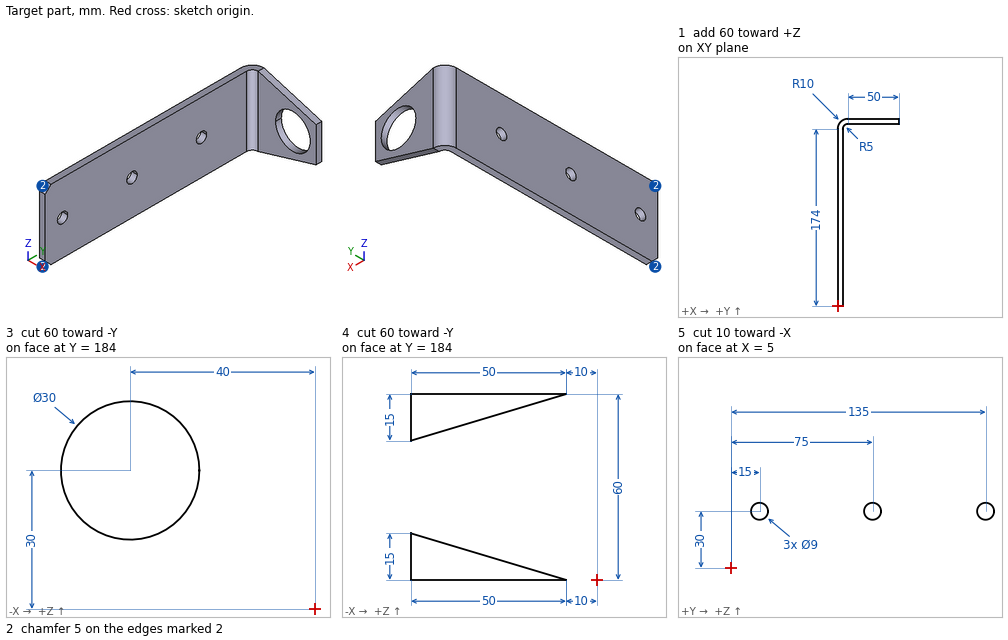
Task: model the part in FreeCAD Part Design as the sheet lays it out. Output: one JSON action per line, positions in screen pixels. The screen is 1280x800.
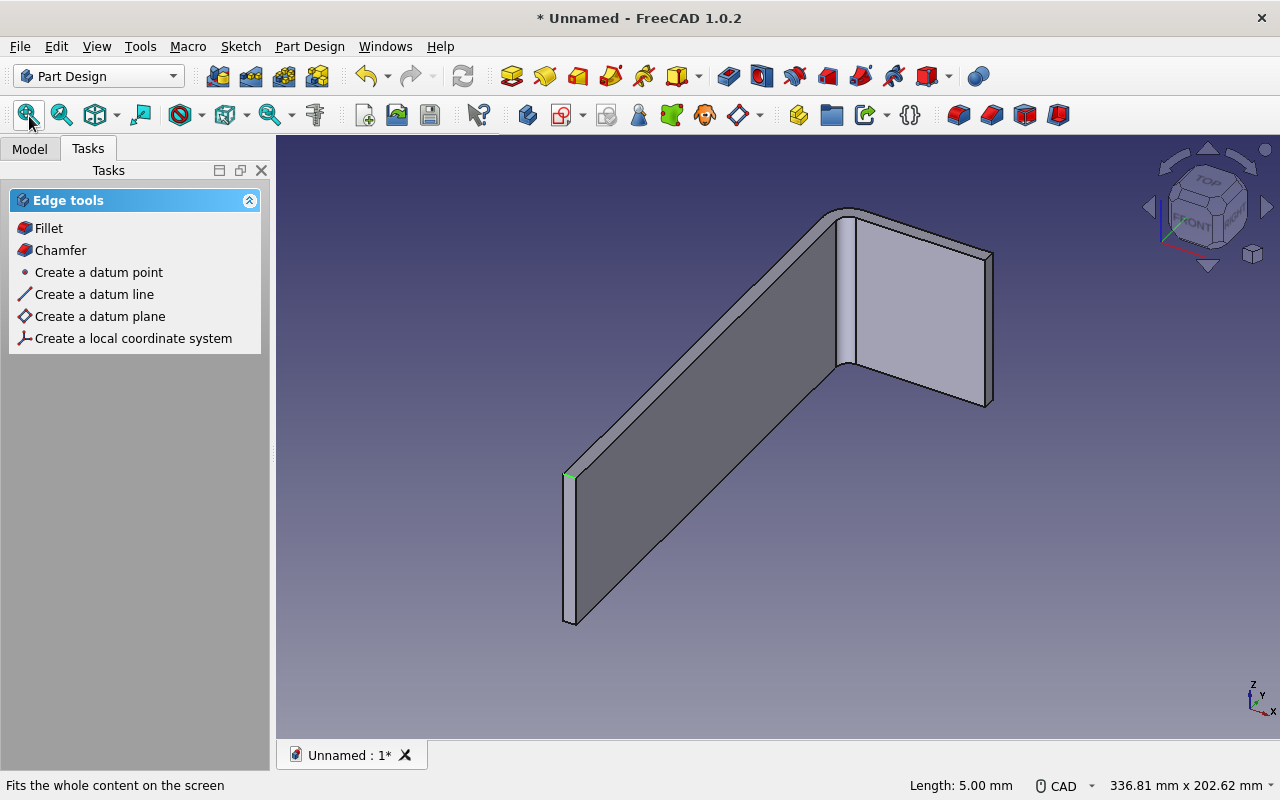
{"action": "key", "text": "0"}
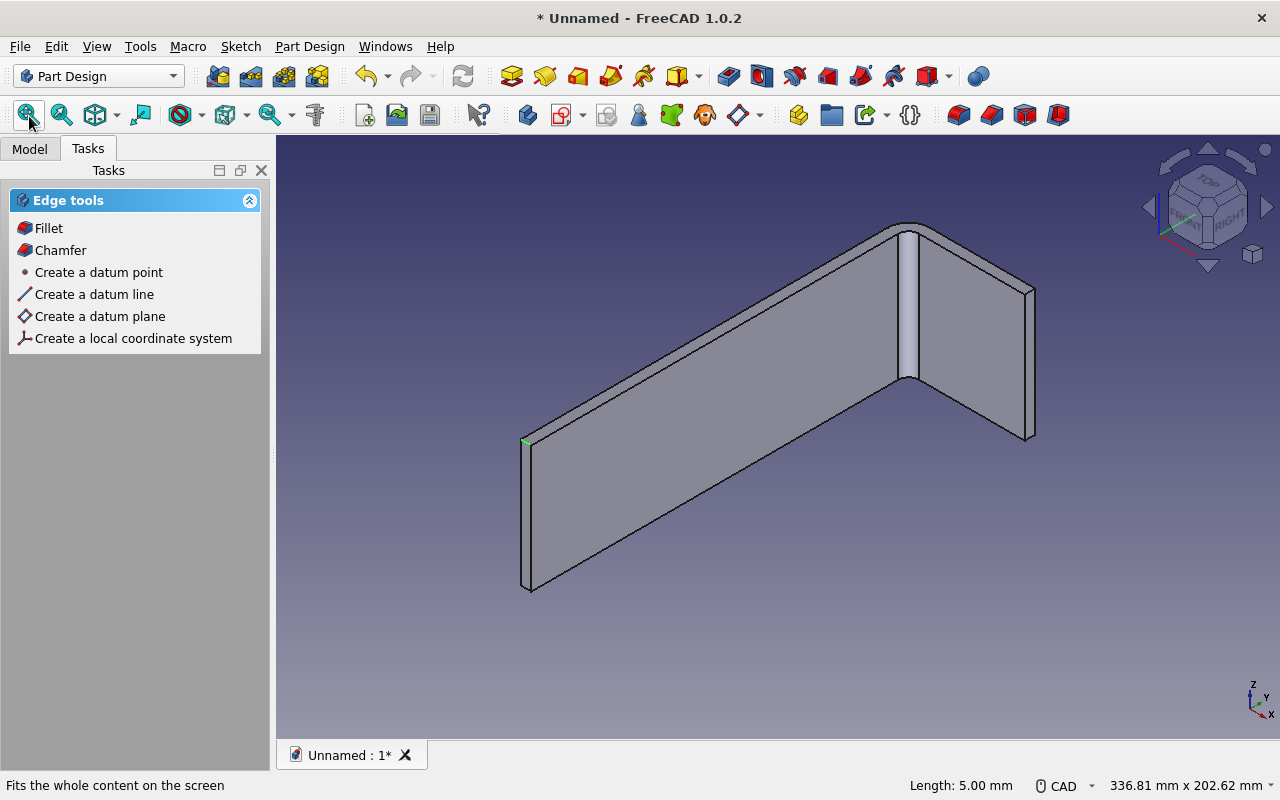
{"action": "scroll", "coordinate": [526, 588], "scroll_direction": "up", "scroll_amount": 5}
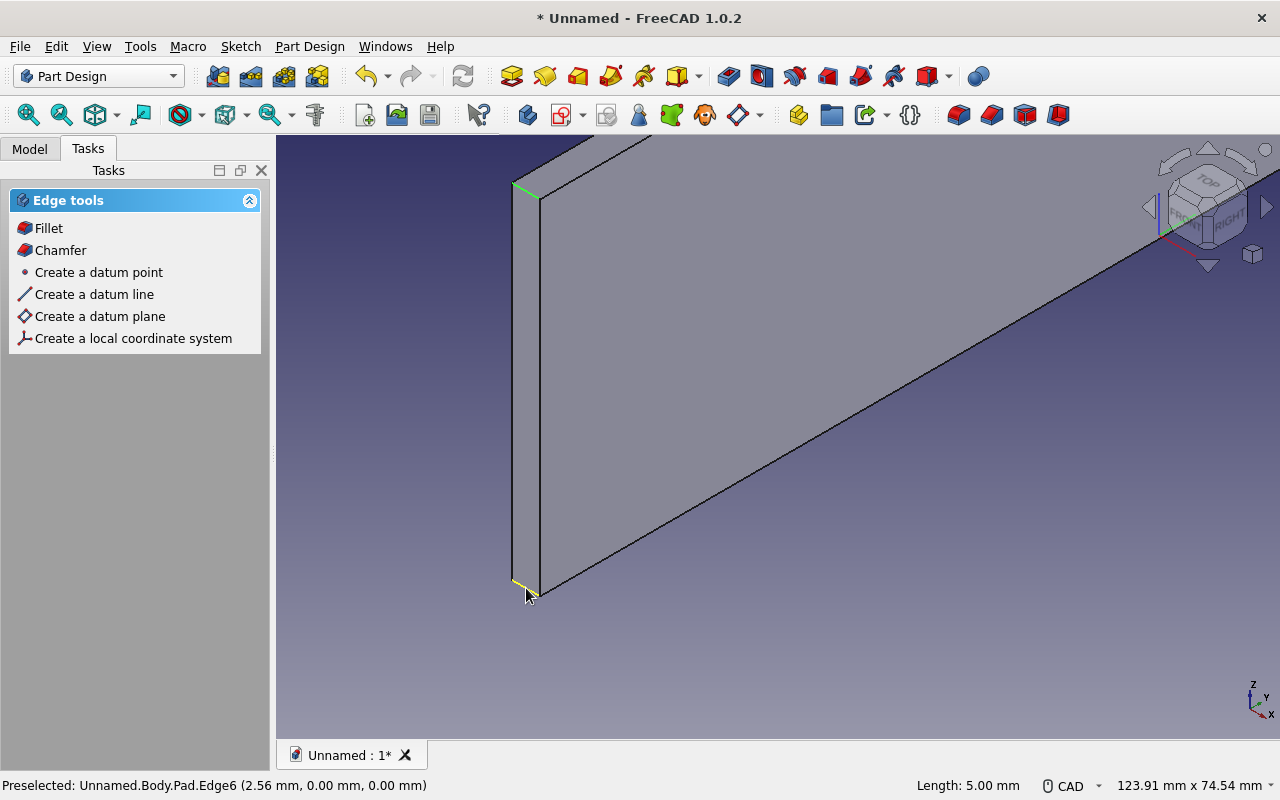
{"action": "key", "text": "v f"}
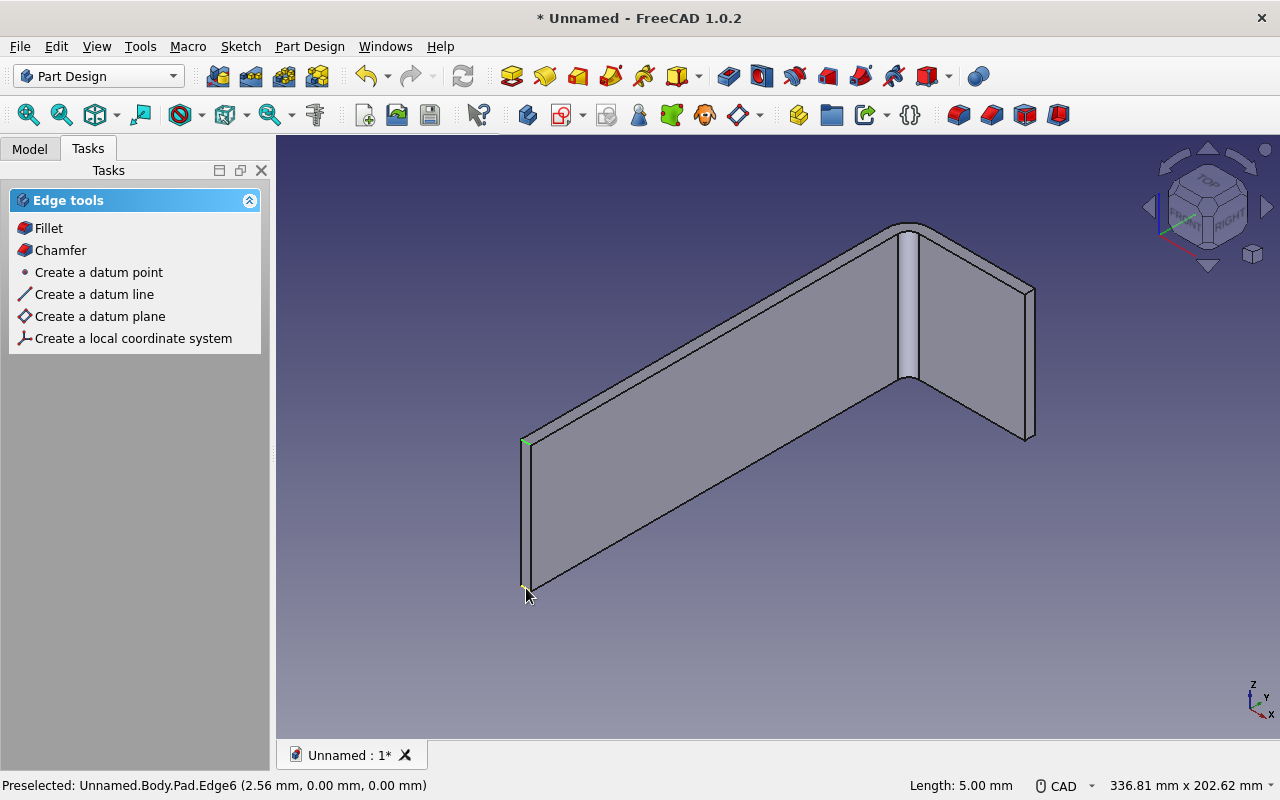
{"action": "key", "text": "2"}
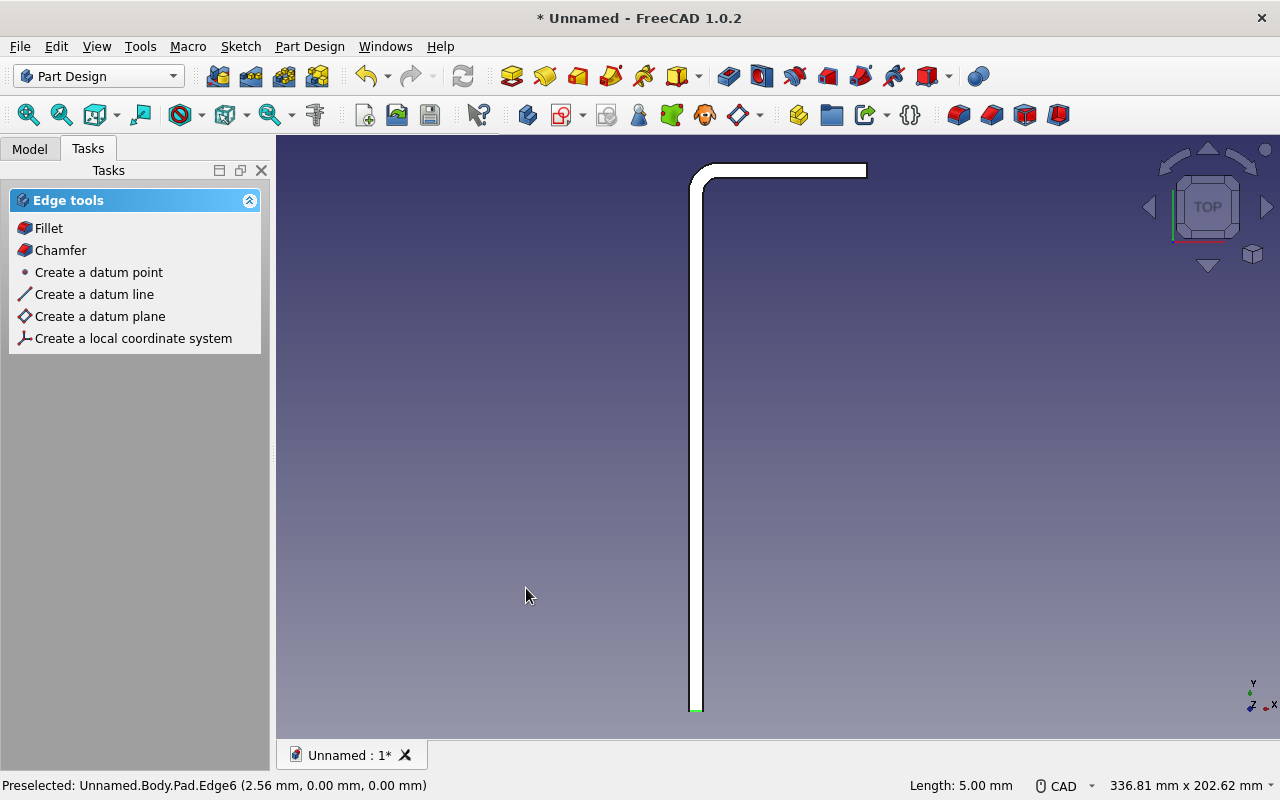
{"action": "scroll", "coordinate": [696, 710], "scroll_direction": "up", "scroll_amount": 5}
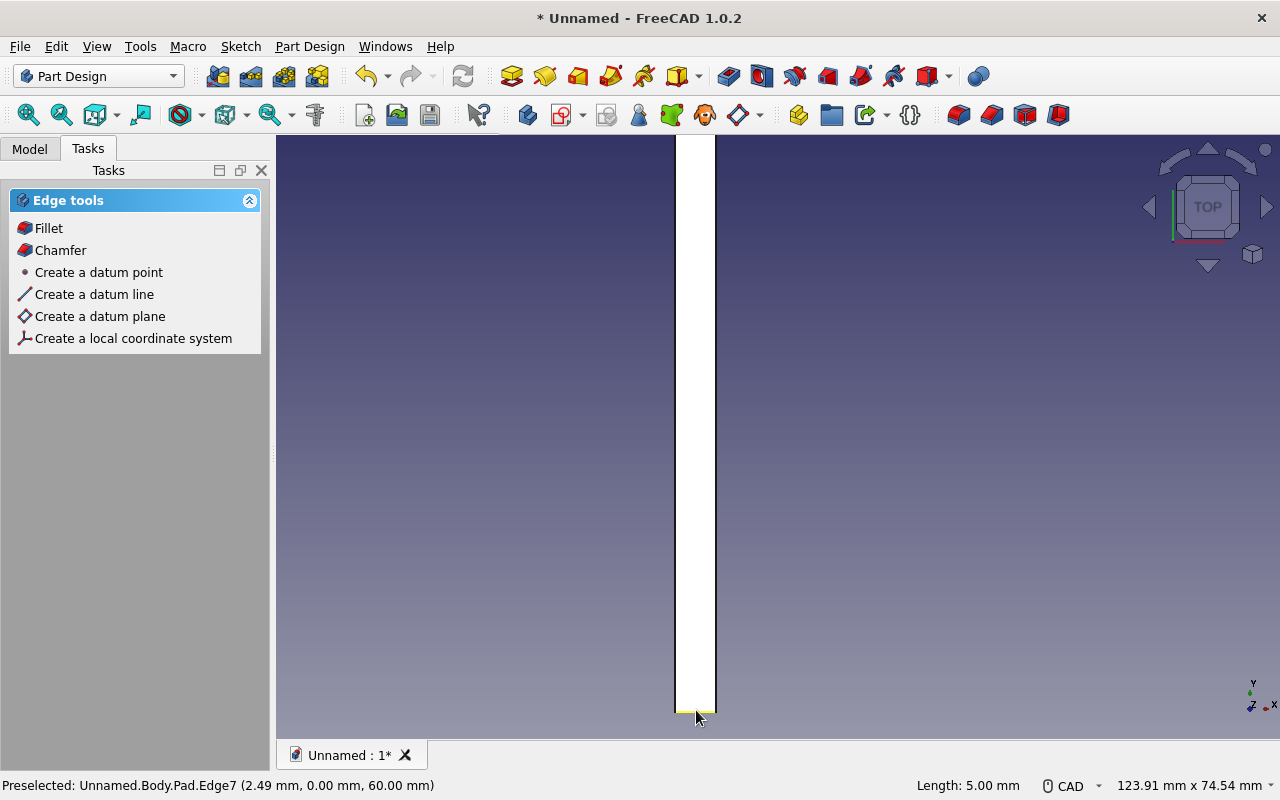
{"action": "key", "text": "v f"}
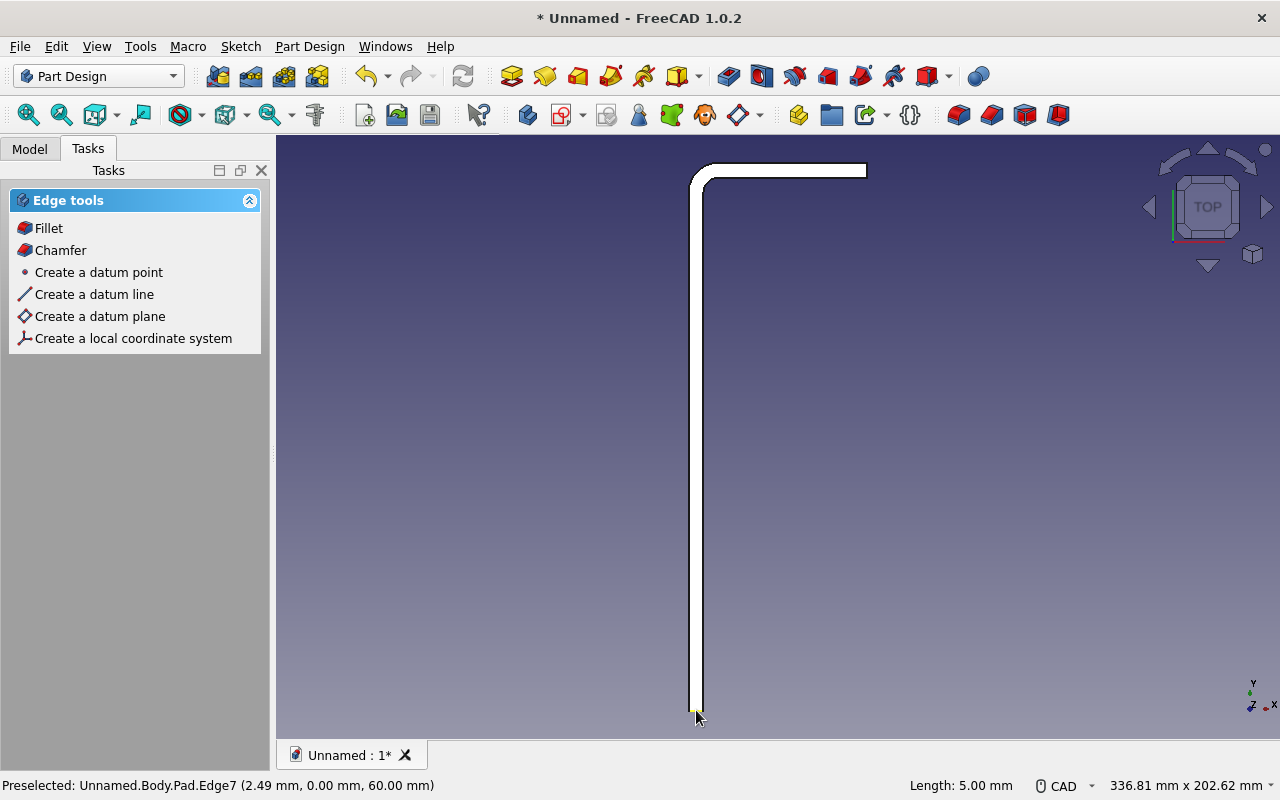
{"action": "key", "text": "1"}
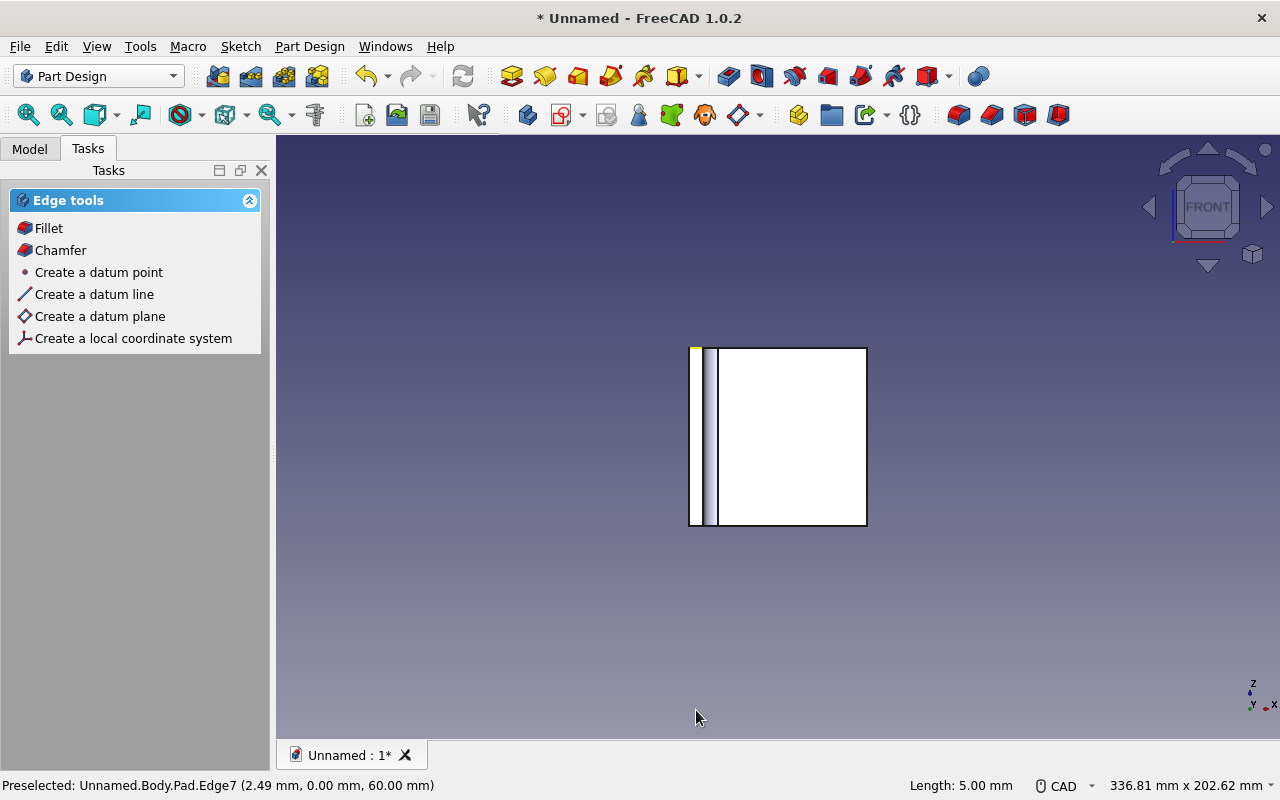
{"action": "key", "text": "v f"}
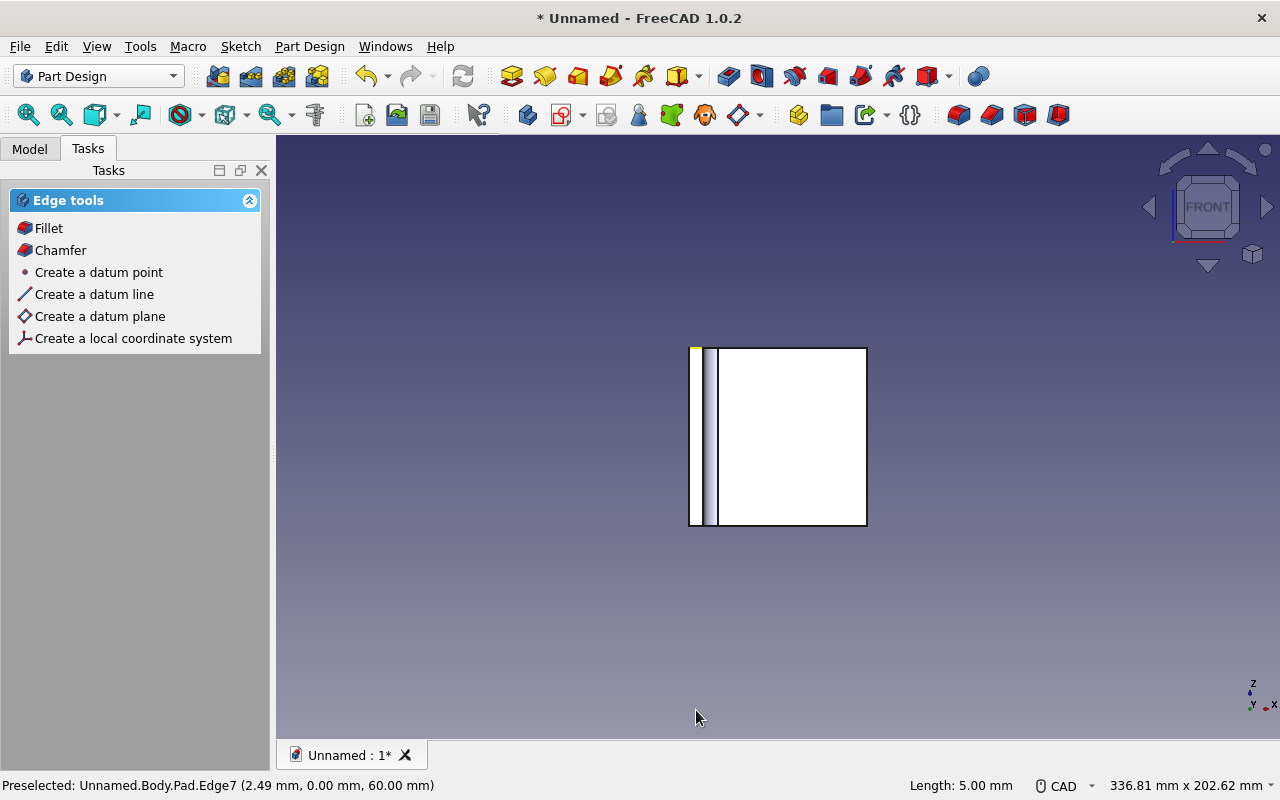
{"action": "left_click", "coordinate": [696, 525], "text": "ctrl"}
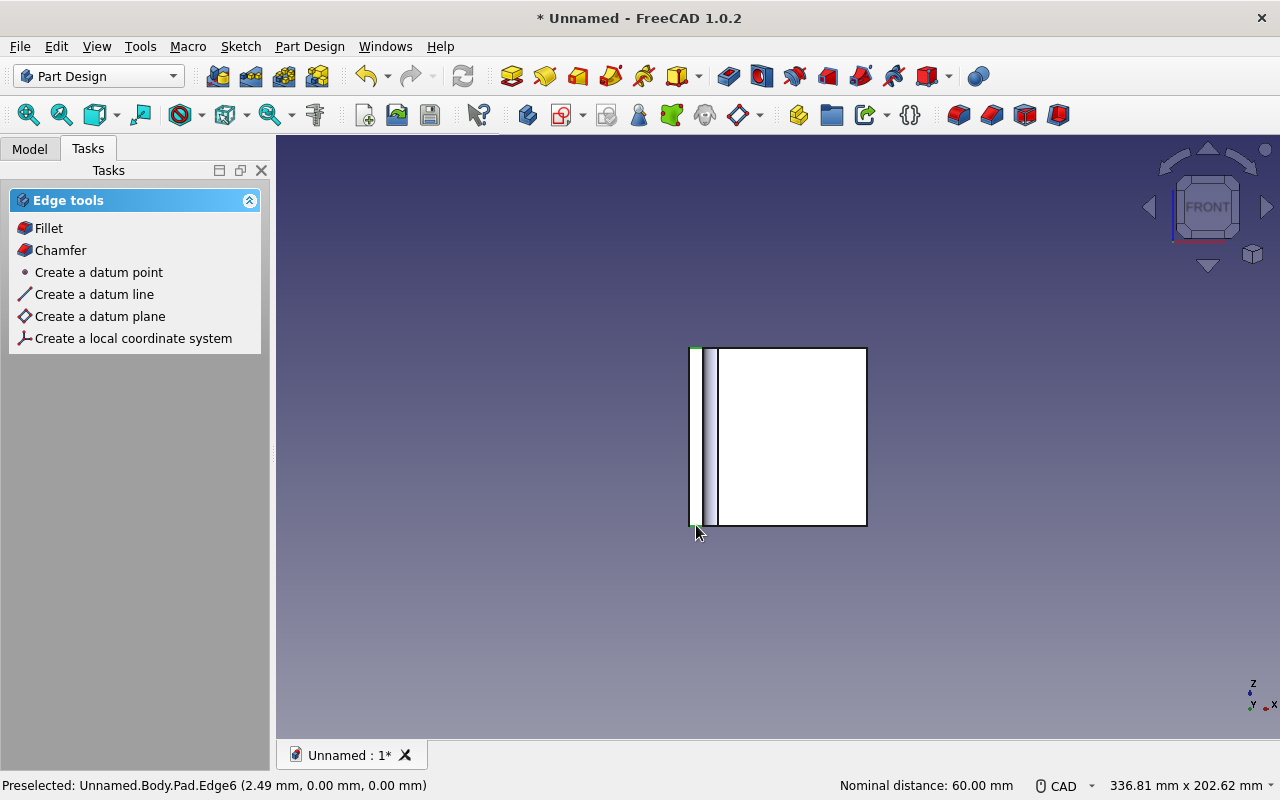
{"action": "left_click", "coordinate": [992, 116]}